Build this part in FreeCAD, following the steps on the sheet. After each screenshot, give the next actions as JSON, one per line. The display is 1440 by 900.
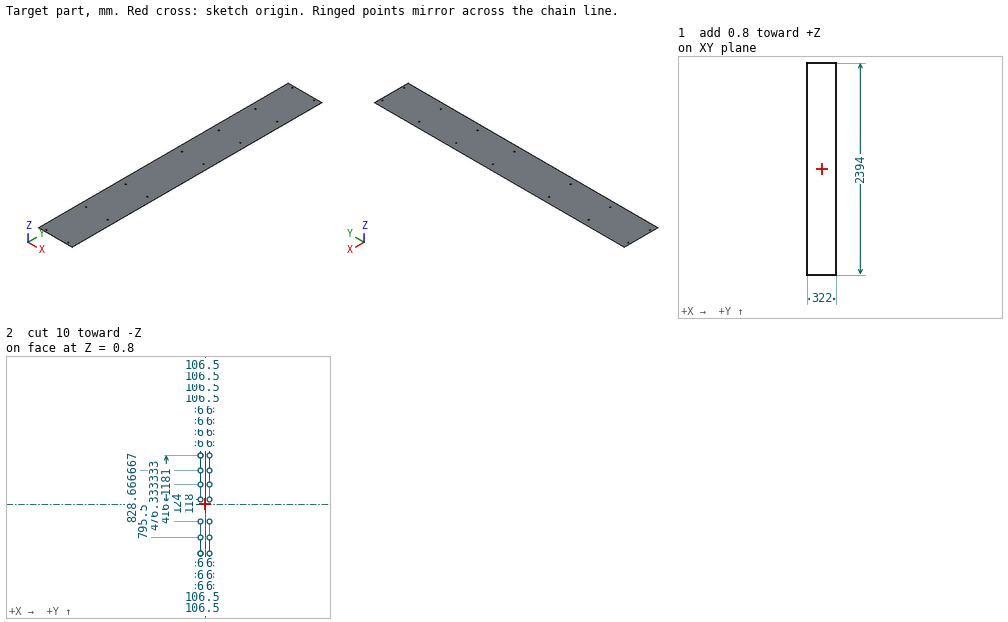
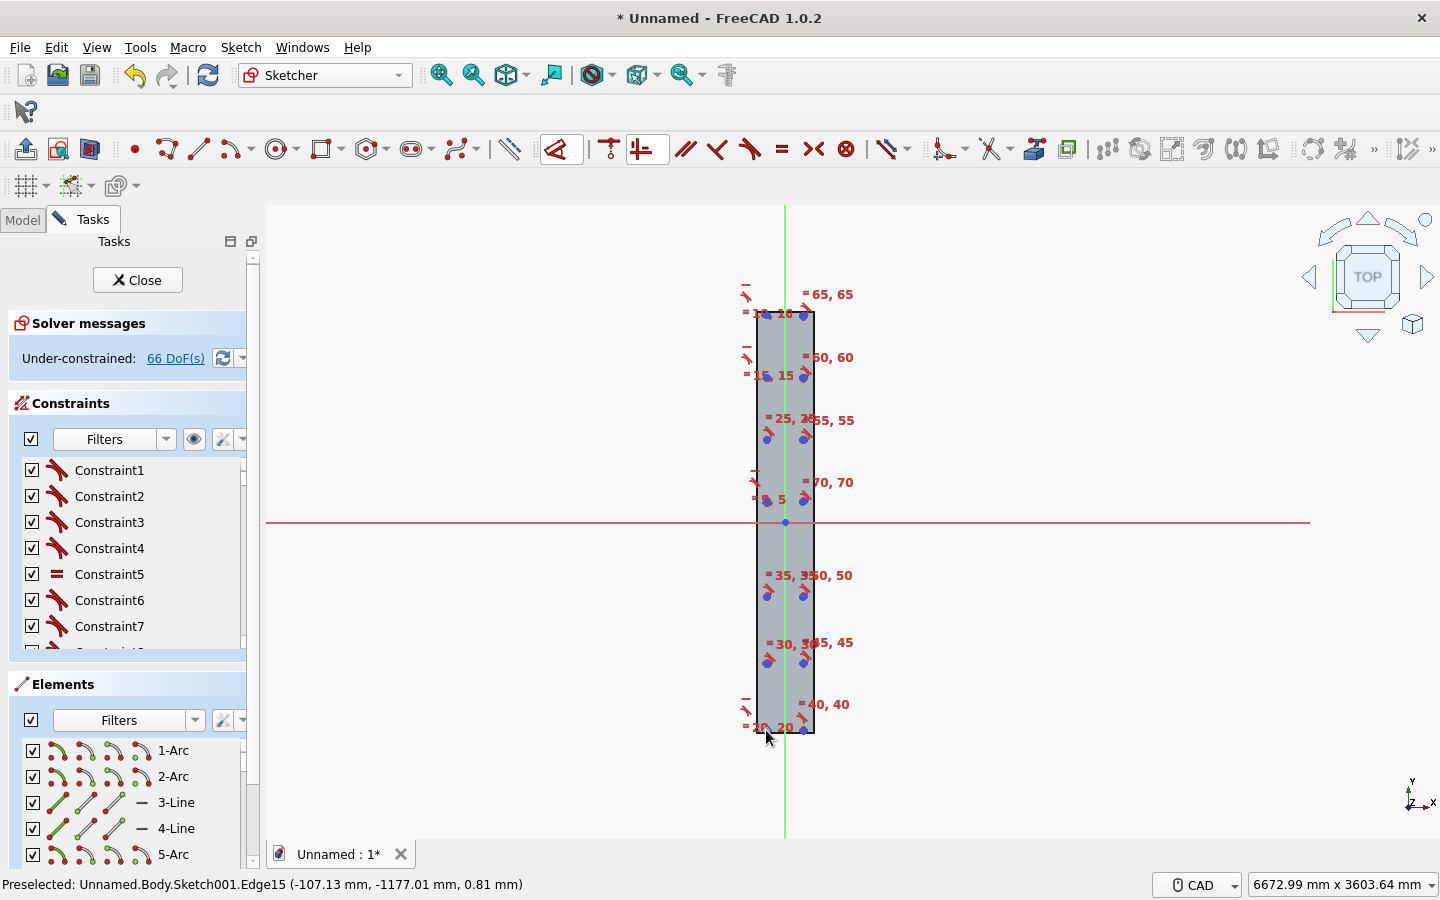
{"action": "scroll", "coordinate": [767, 439], "scroll_direction": "up", "scroll_amount": 14}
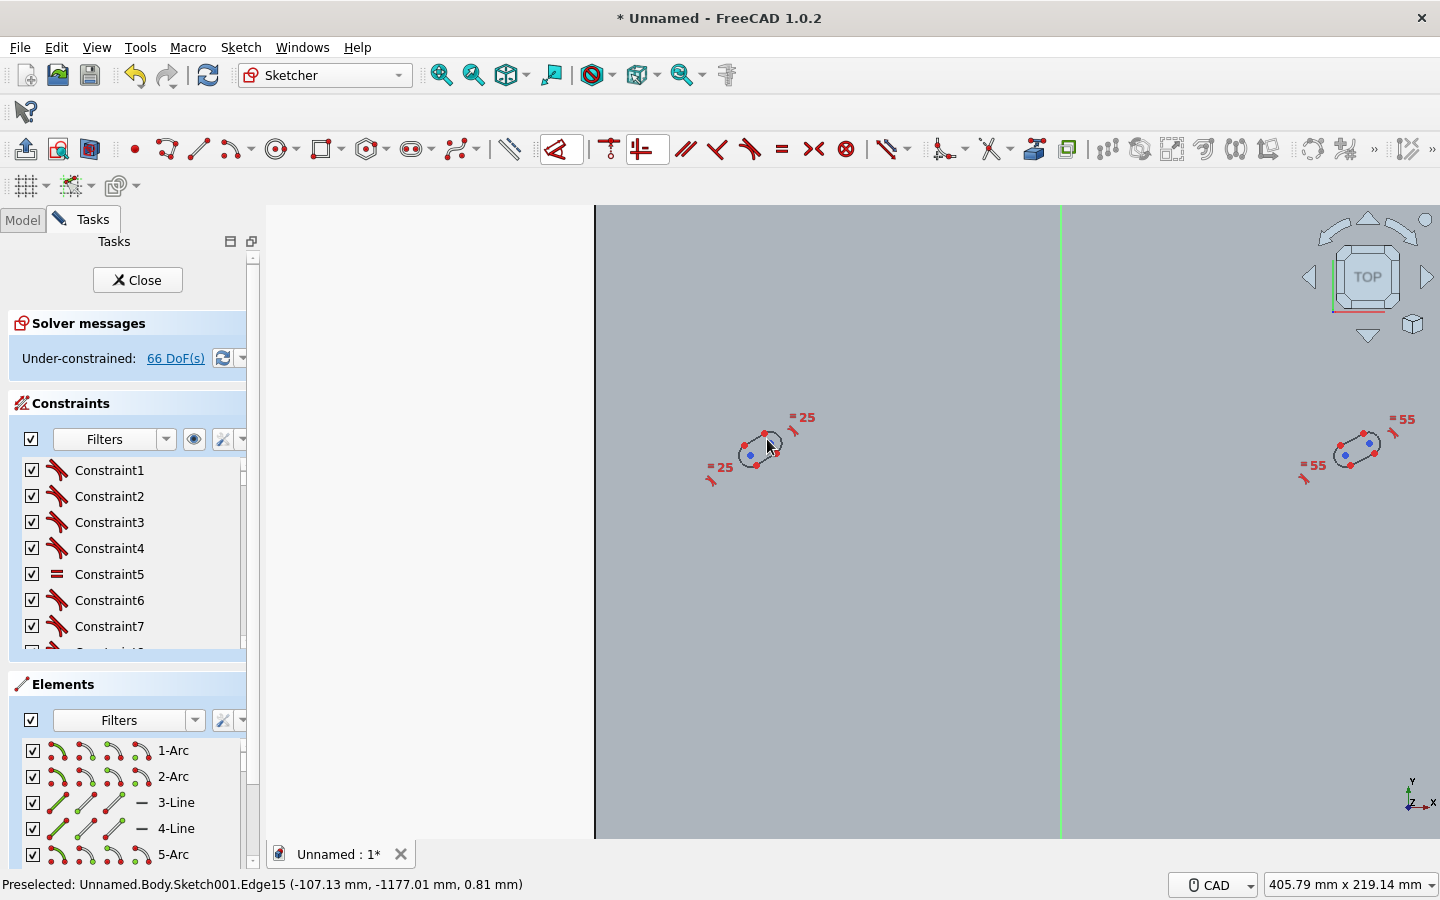
{"action": "left_click", "coordinate": [752, 441]}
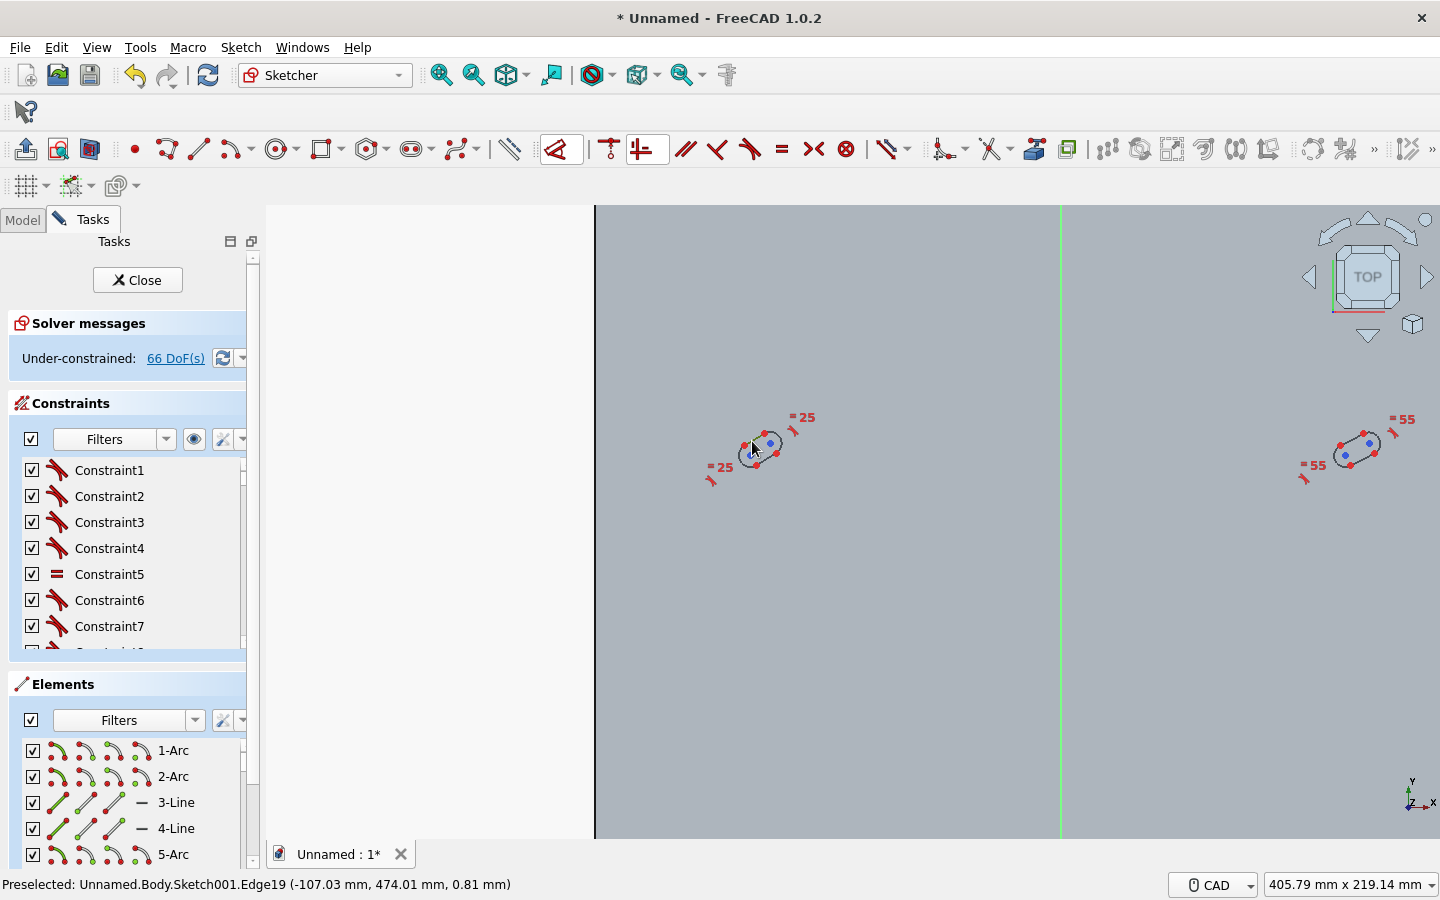
{"action": "key", "text": "h"}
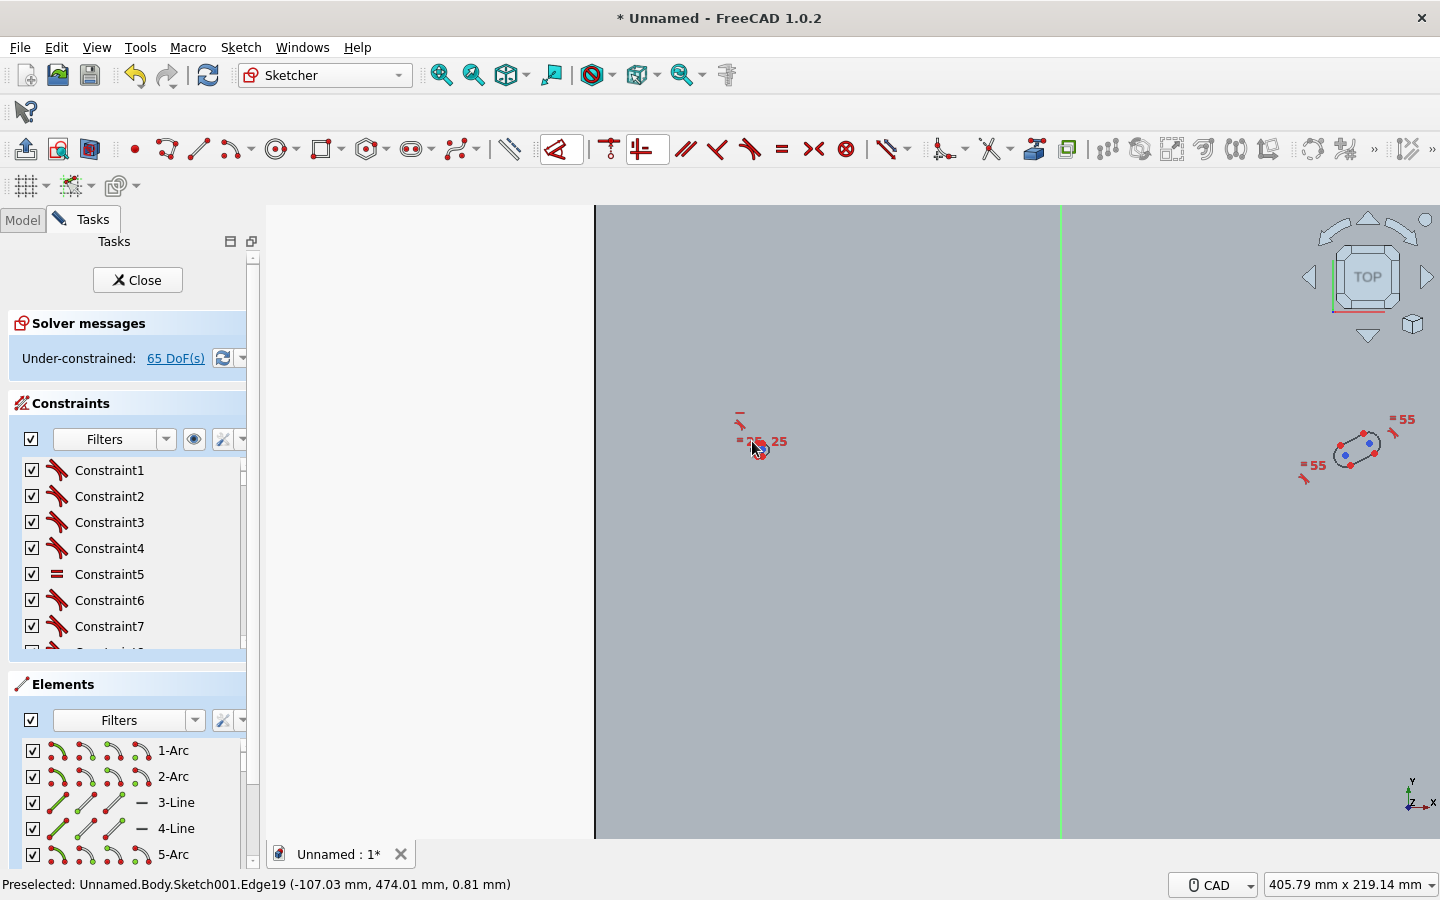
{"action": "scroll", "coordinate": [767, 438], "scroll_direction": "down", "scroll_amount": 14}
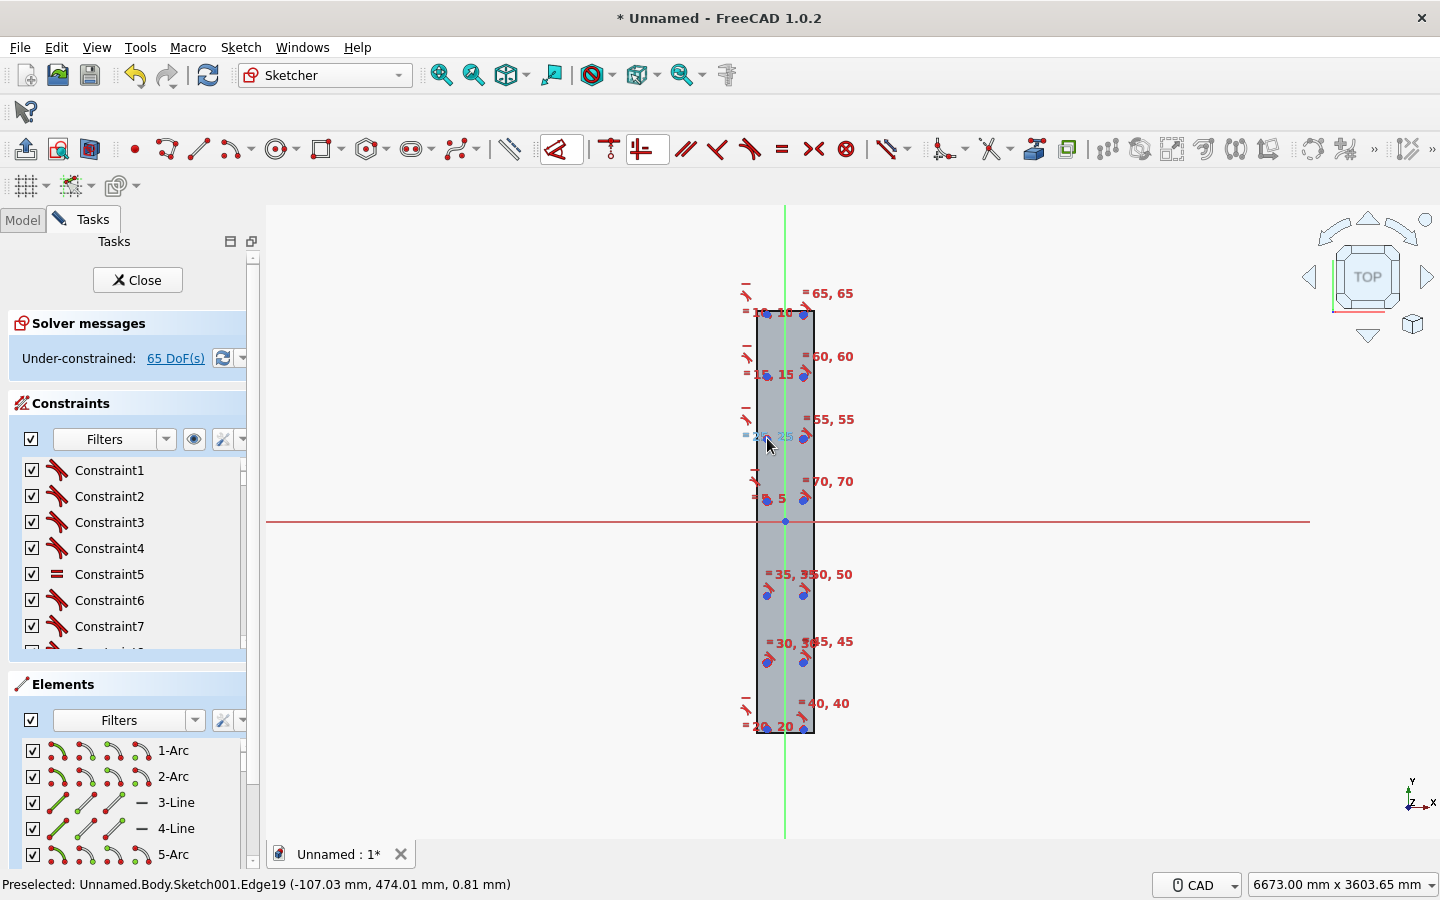
{"action": "scroll", "coordinate": [766, 662], "scroll_direction": "up", "scroll_amount": 14}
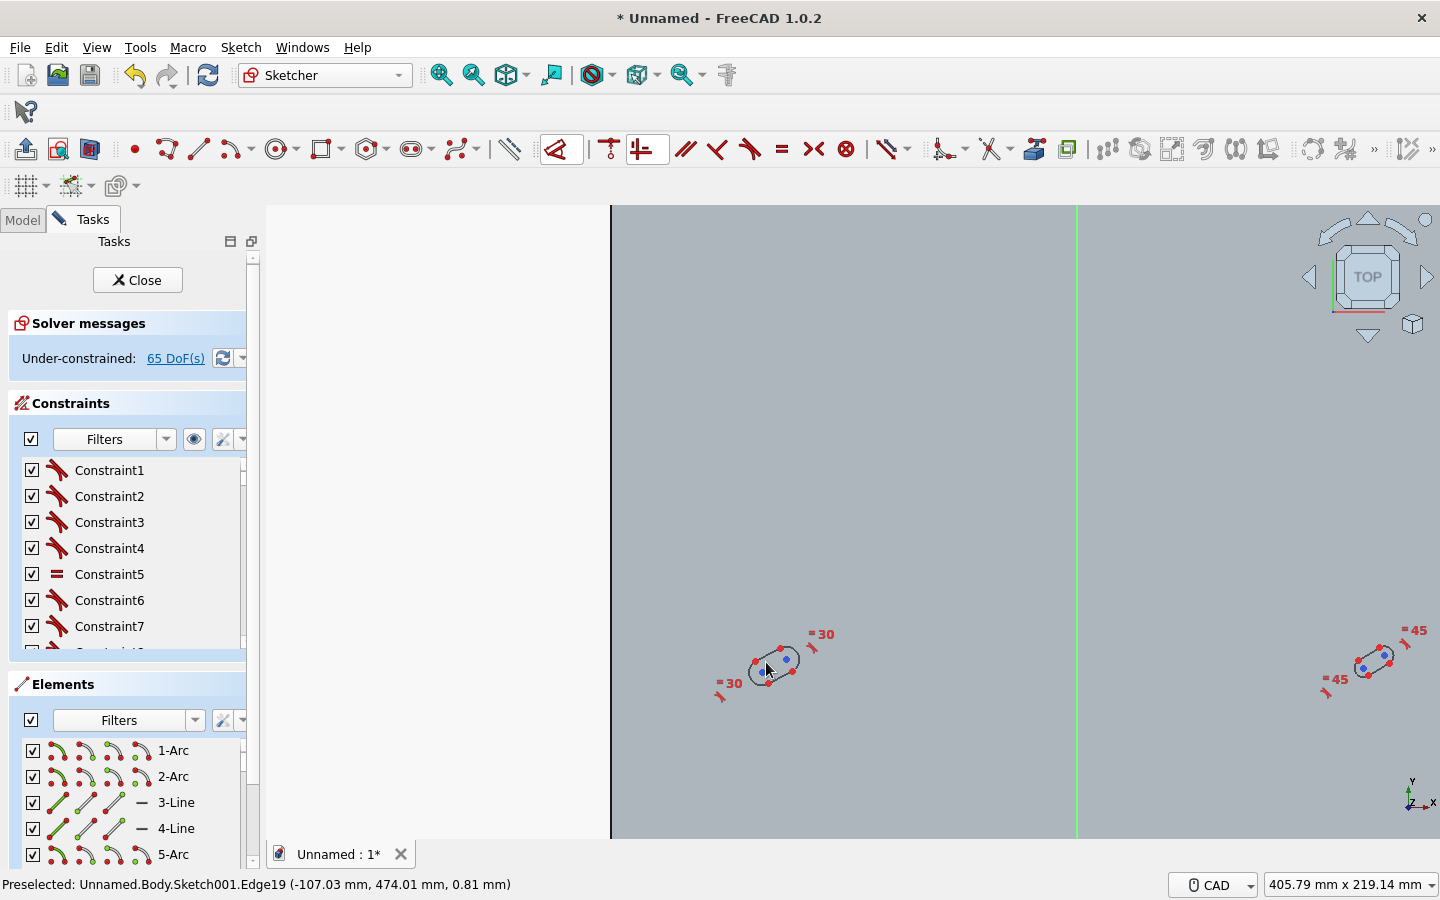
{"action": "left_click", "coordinate": [766, 656]}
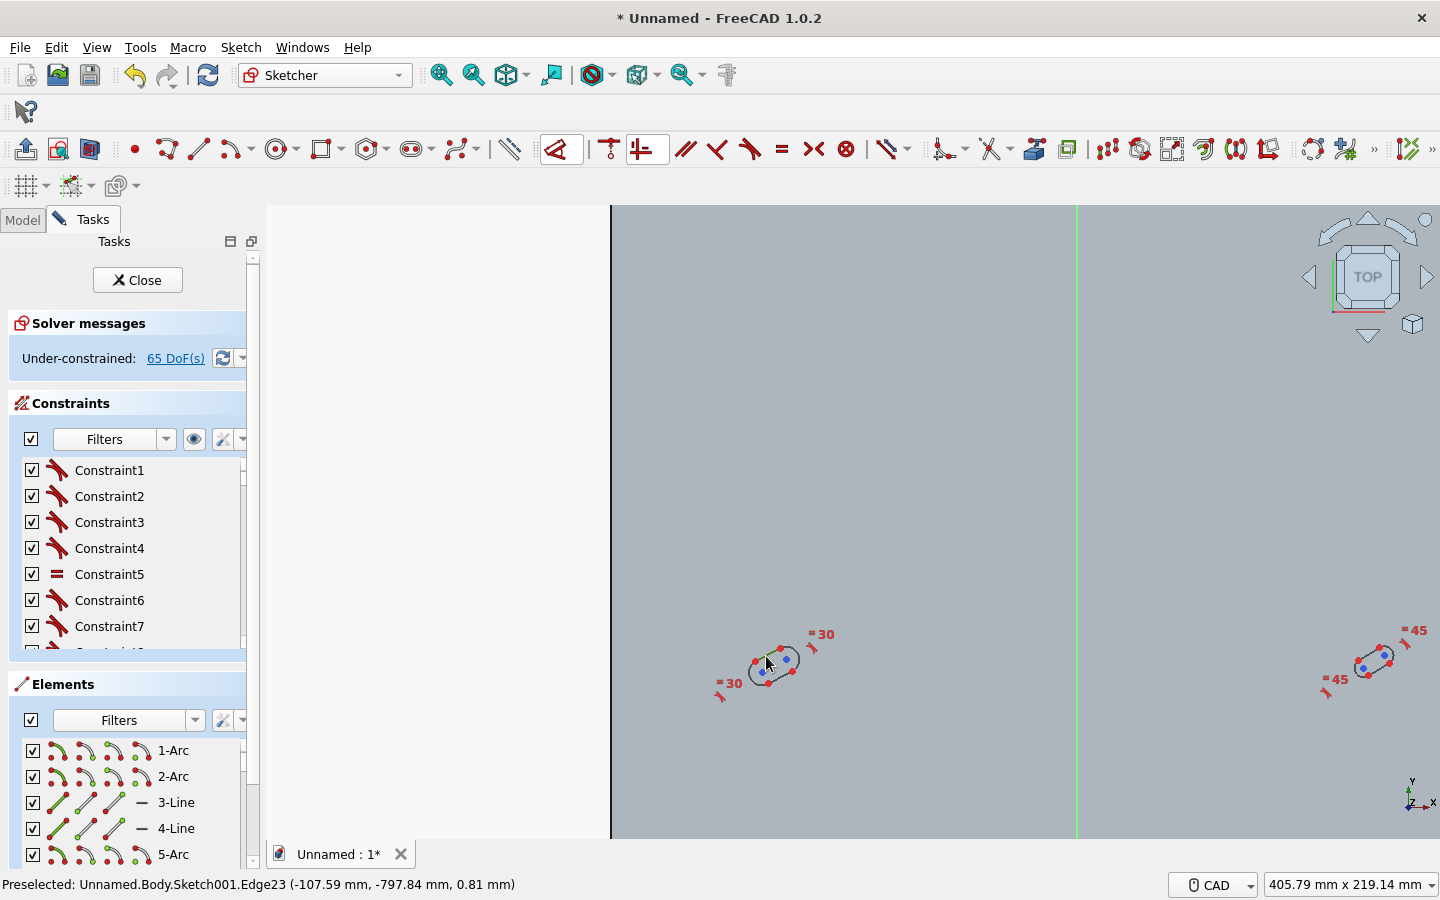
{"action": "key", "text": "h"}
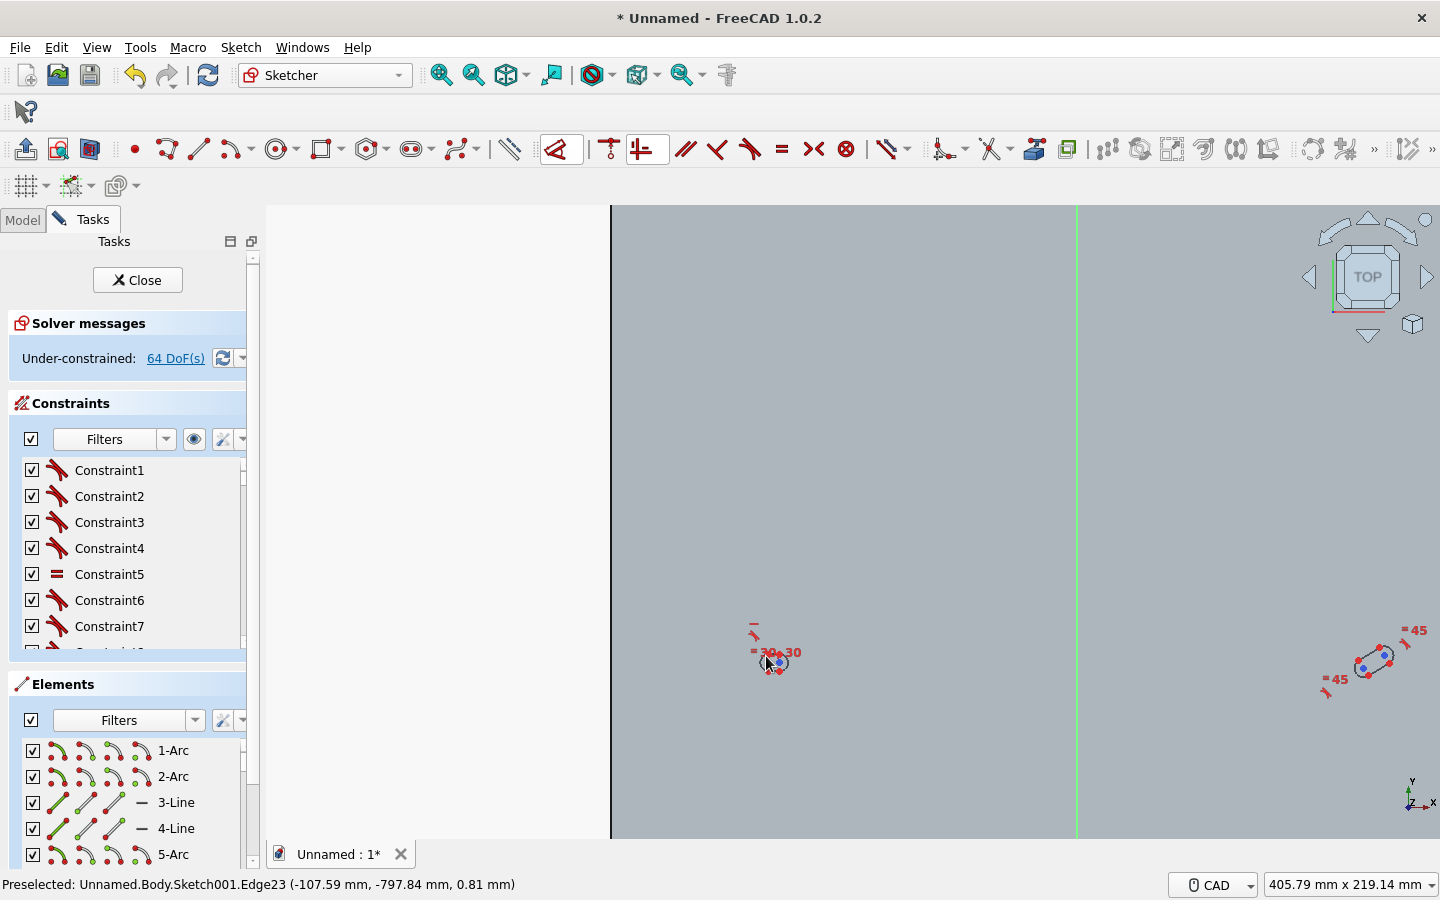
{"action": "scroll", "coordinate": [766, 663], "scroll_direction": "down", "scroll_amount": 14}